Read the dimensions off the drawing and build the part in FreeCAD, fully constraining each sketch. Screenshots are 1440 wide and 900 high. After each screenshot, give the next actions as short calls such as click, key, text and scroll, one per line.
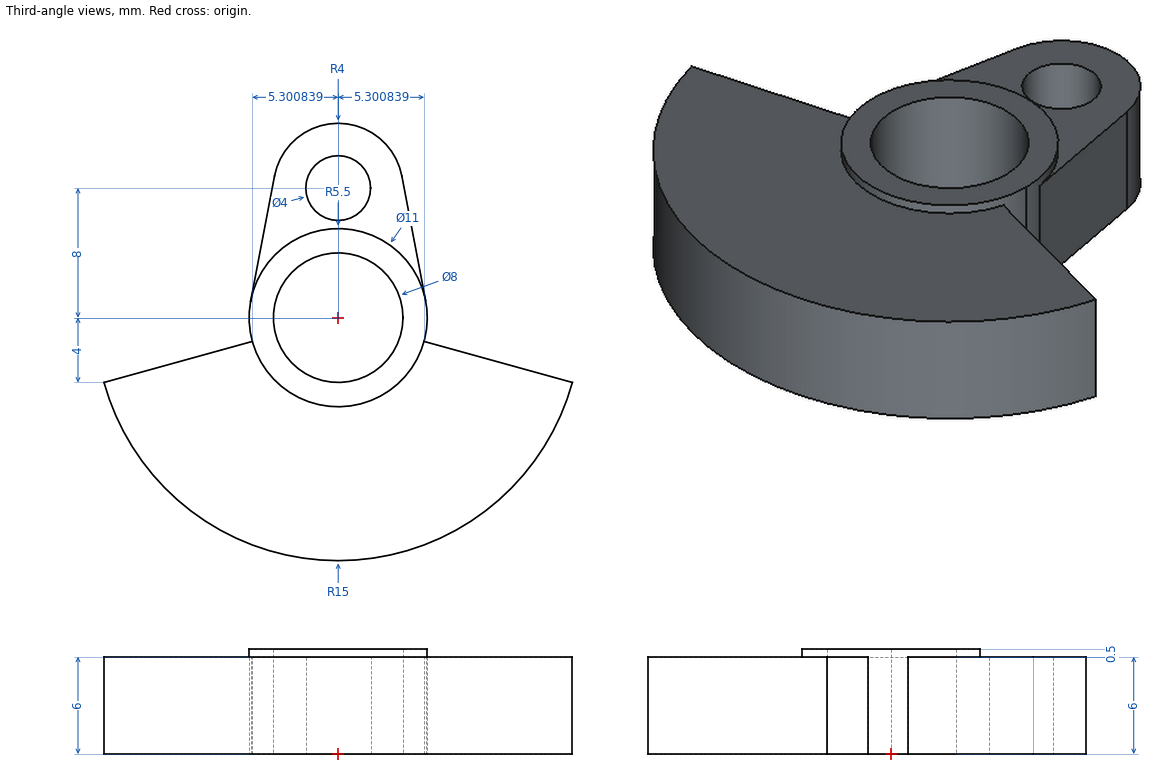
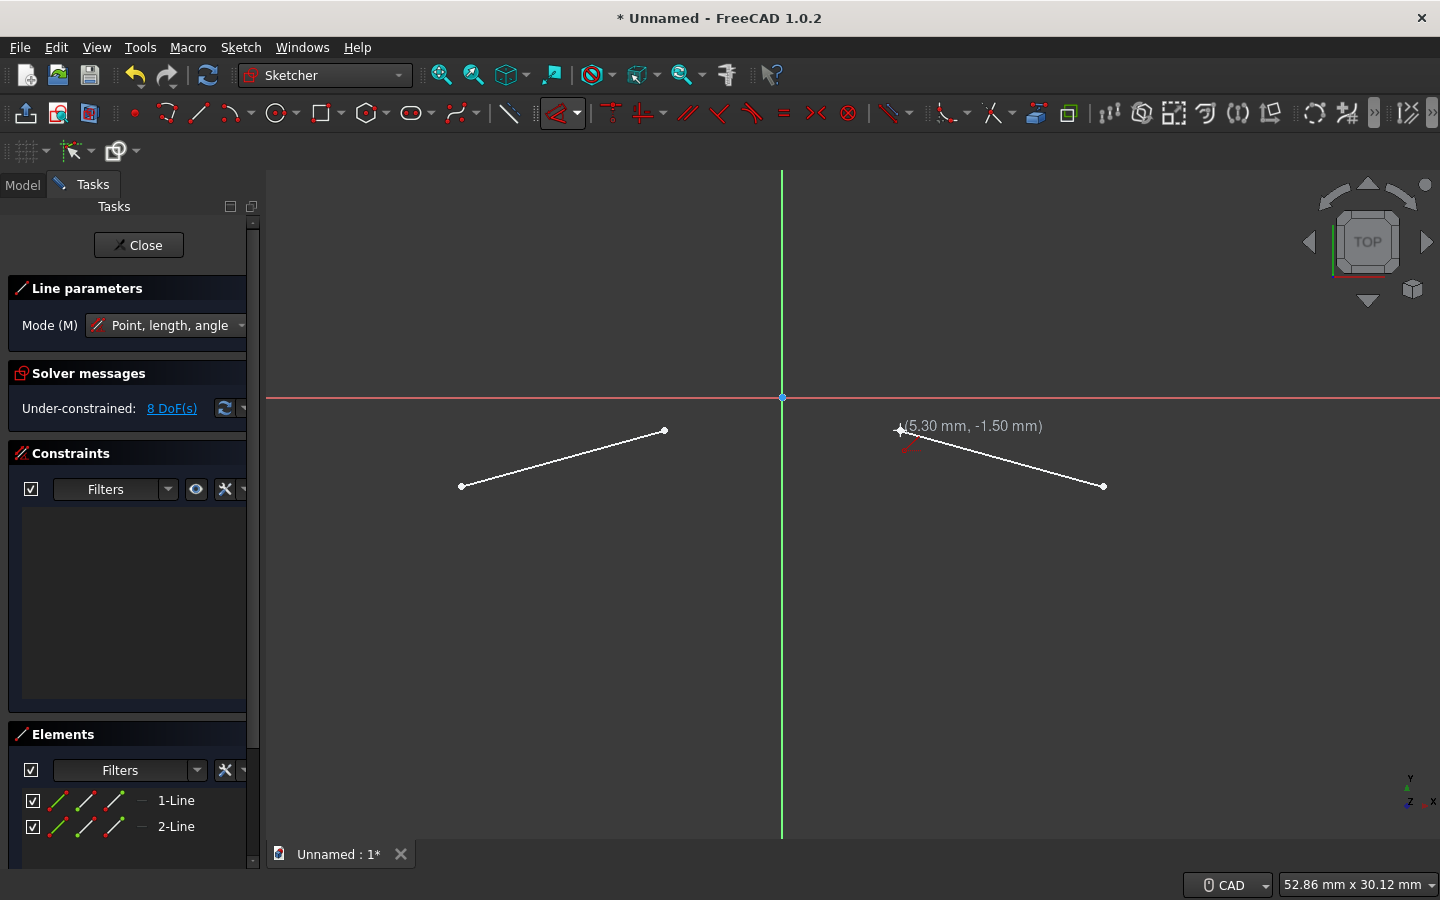
key(g)
key(3)
key(a)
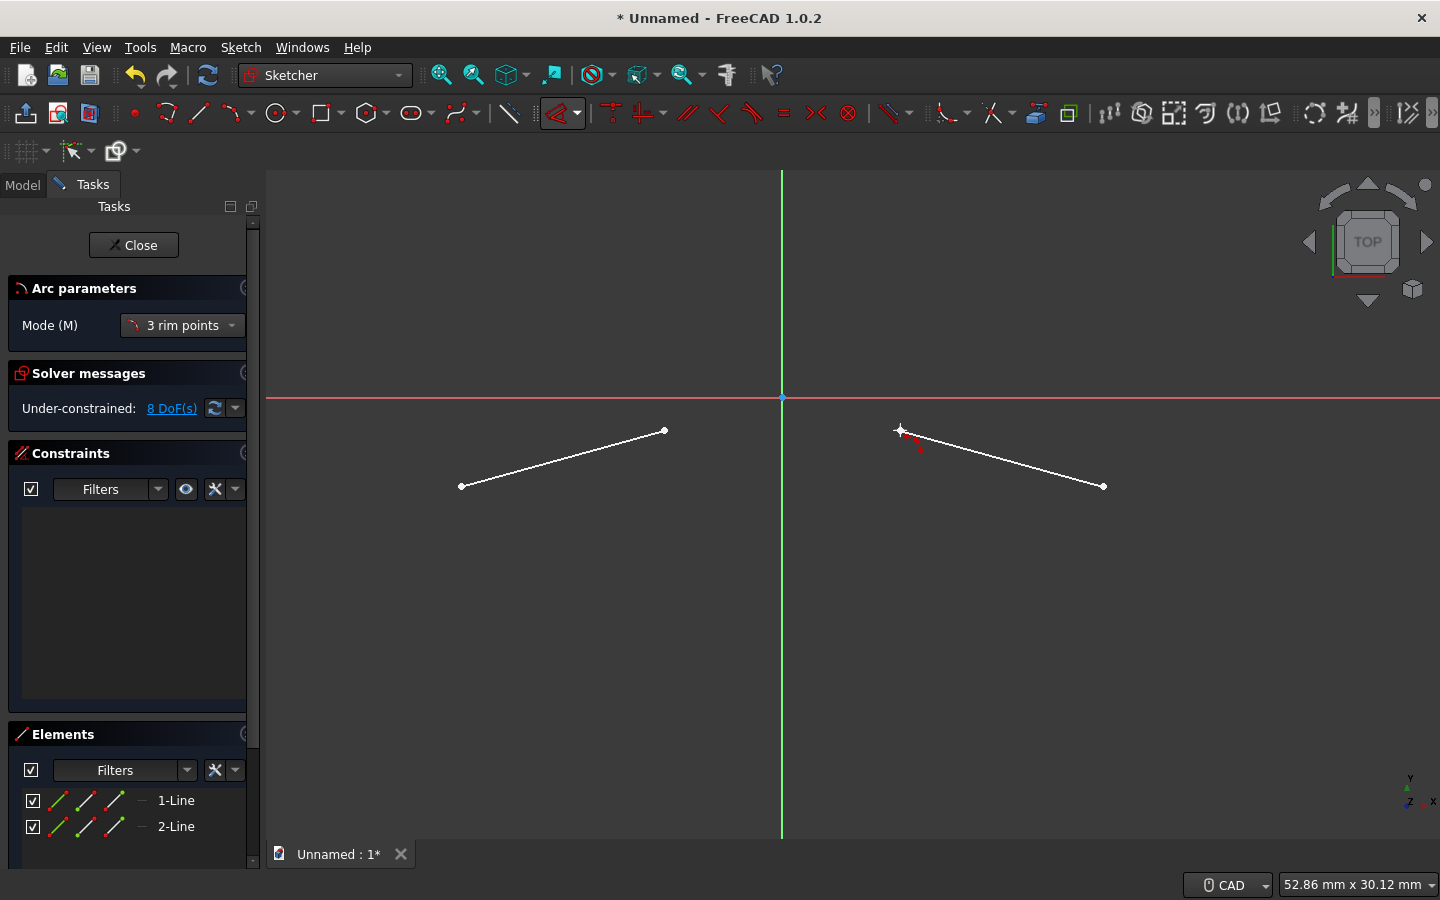
click(461, 487)
click(1103, 487)
click(696, 720)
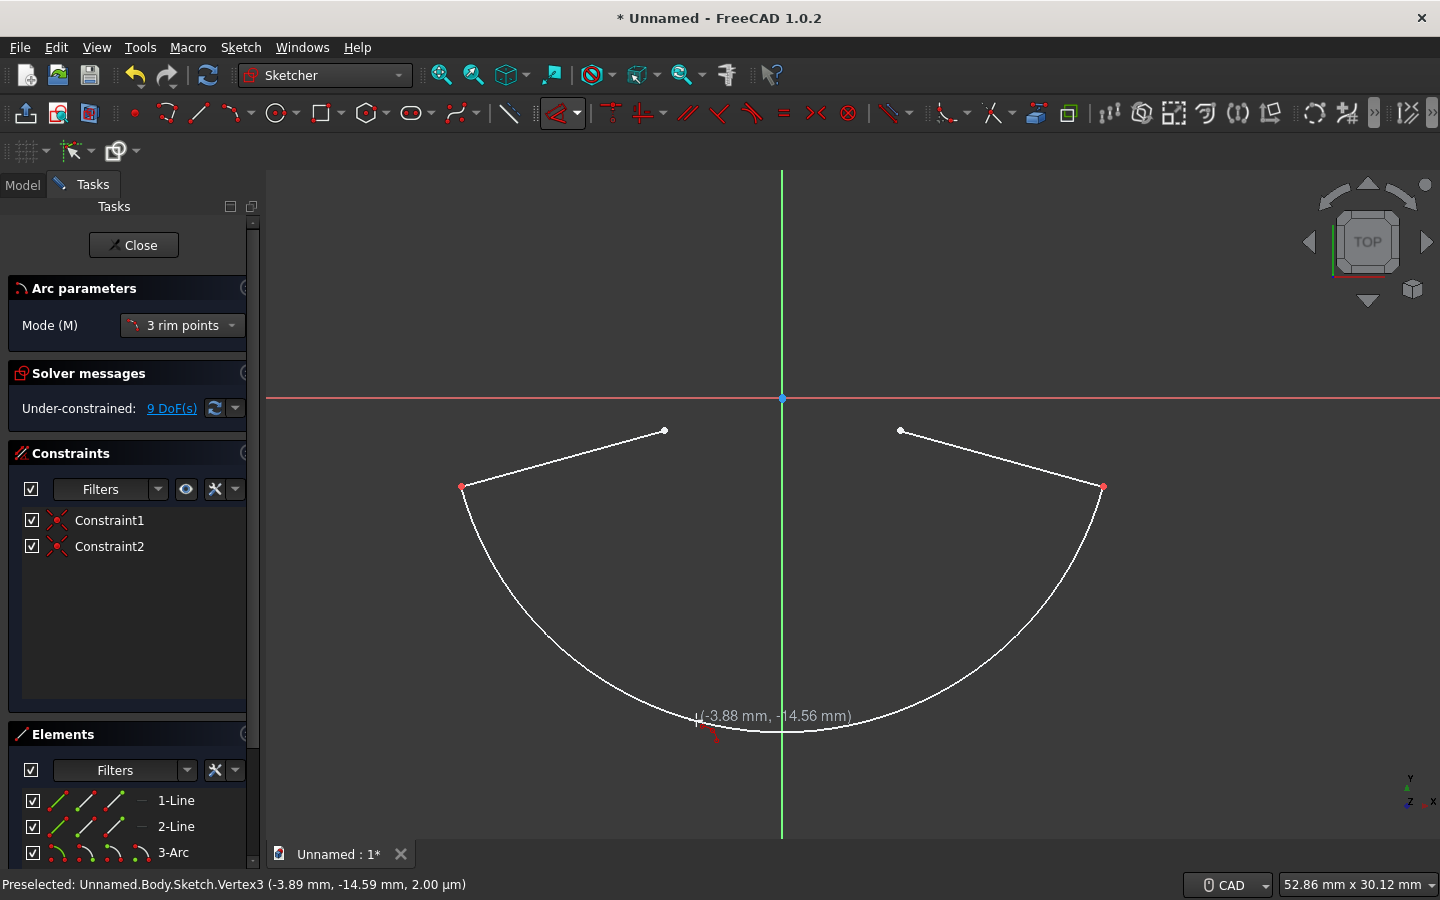
click(900, 431)
click(664, 431)
click(826, 284)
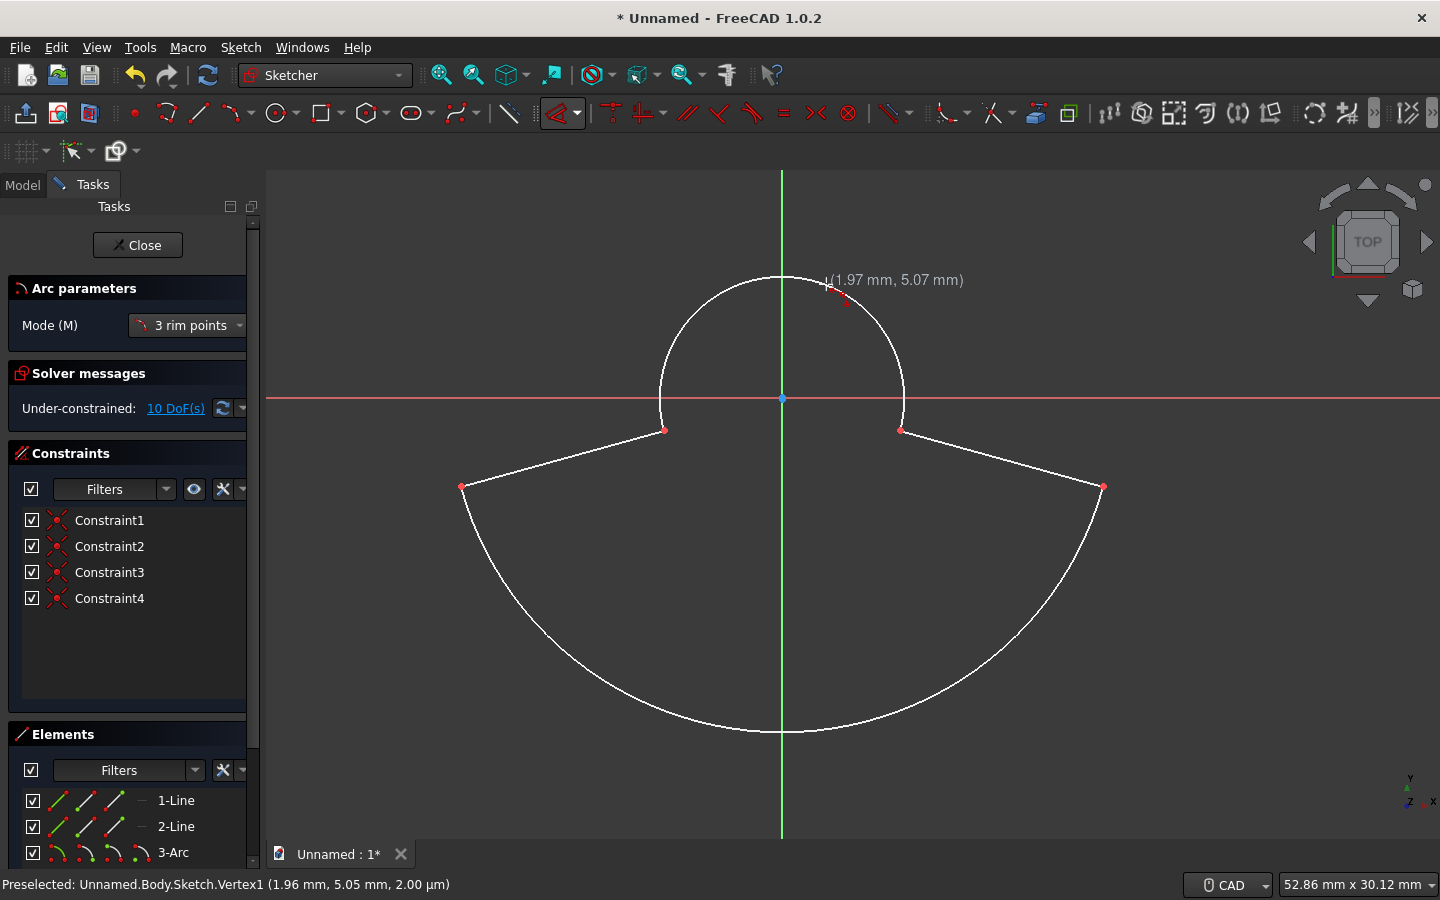
click(276, 114)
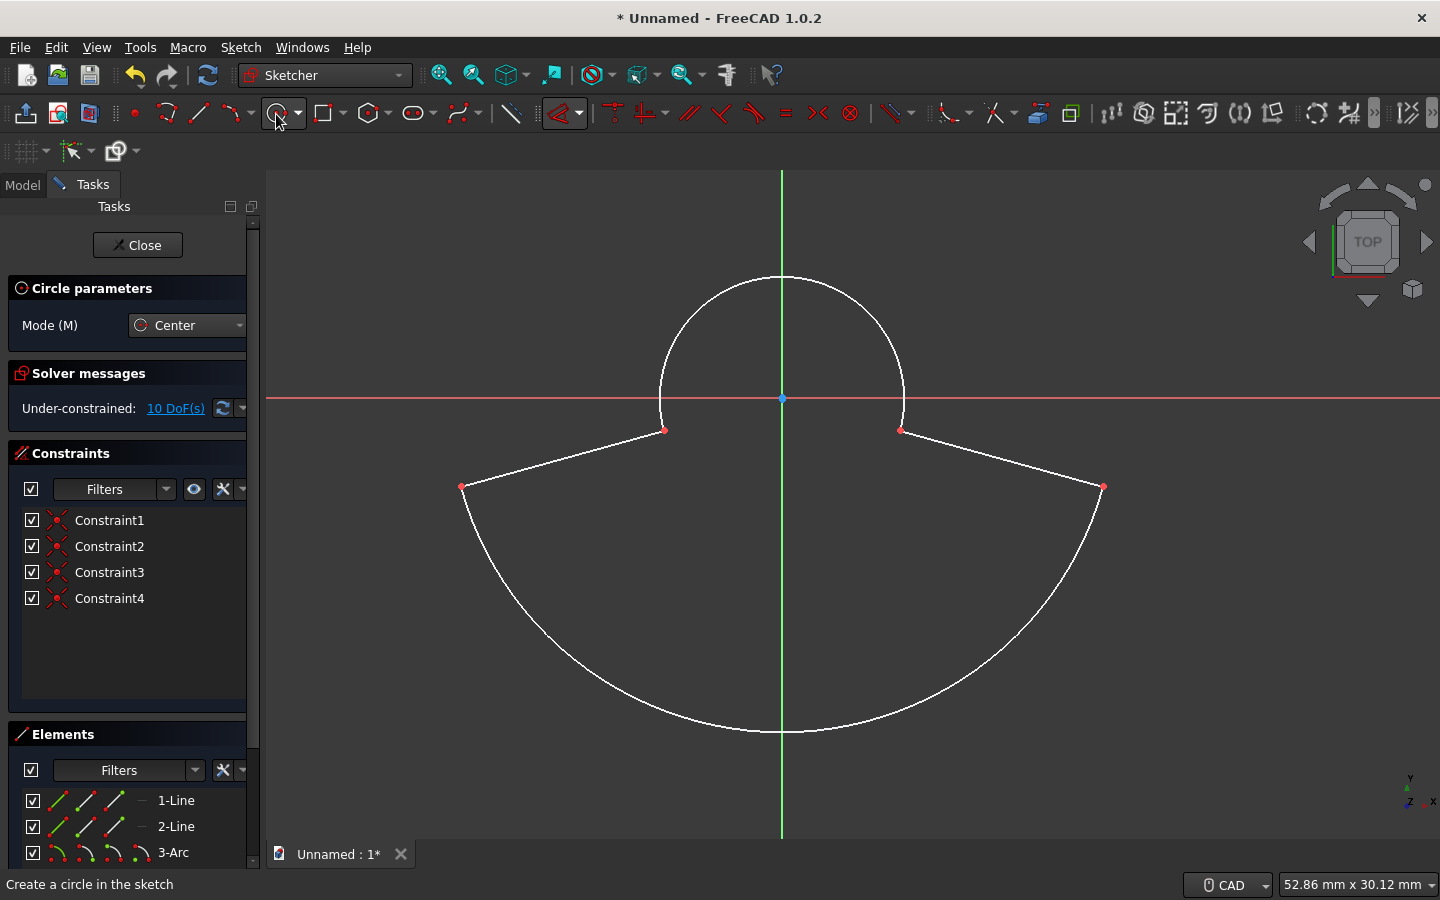
click(782, 398)
click(845, 335)
key(Escape)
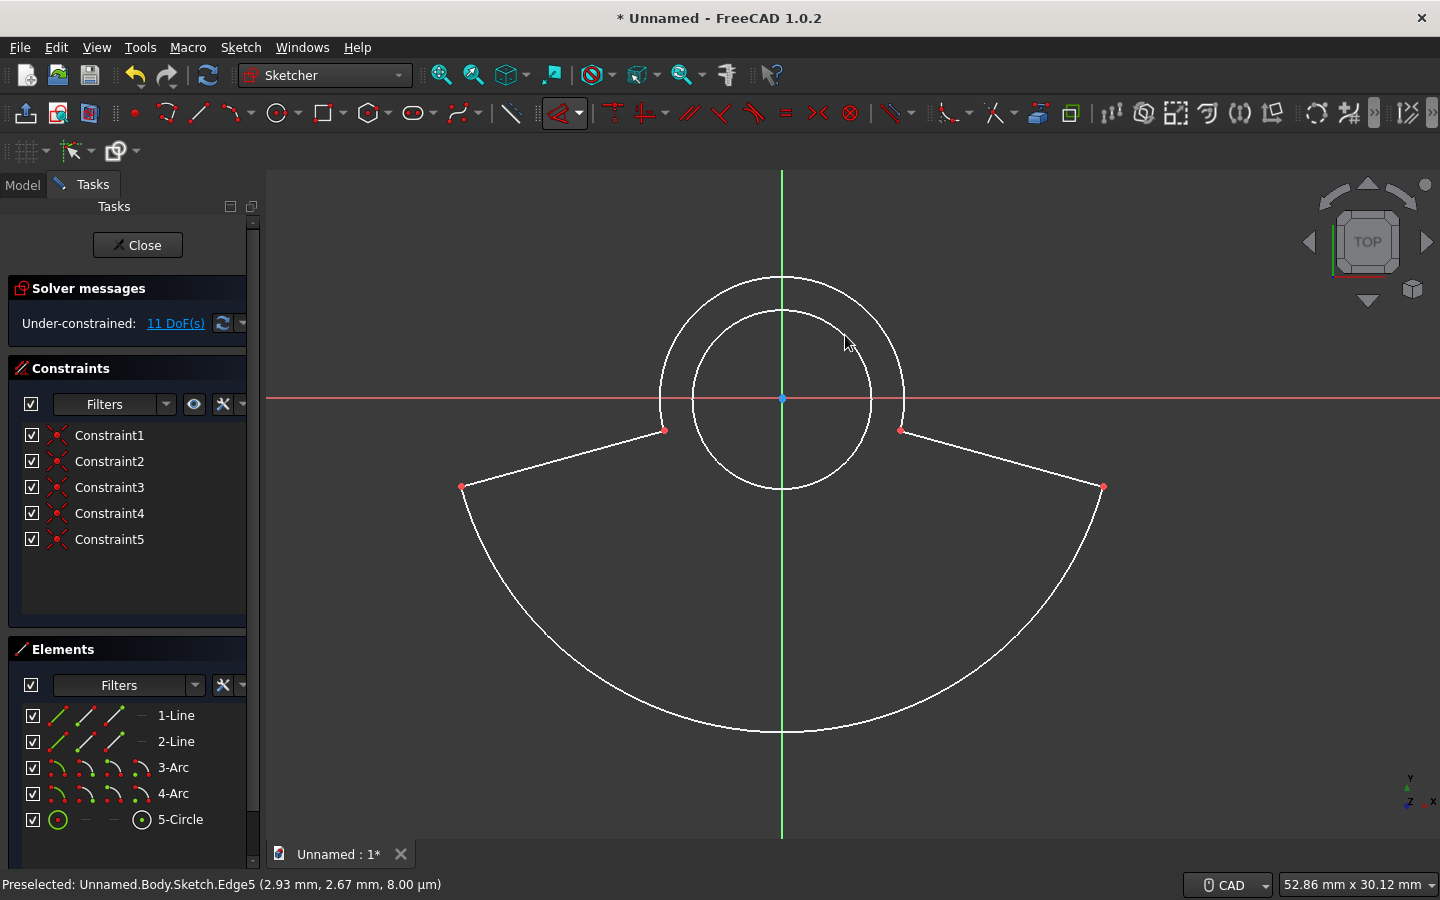
click(845, 336)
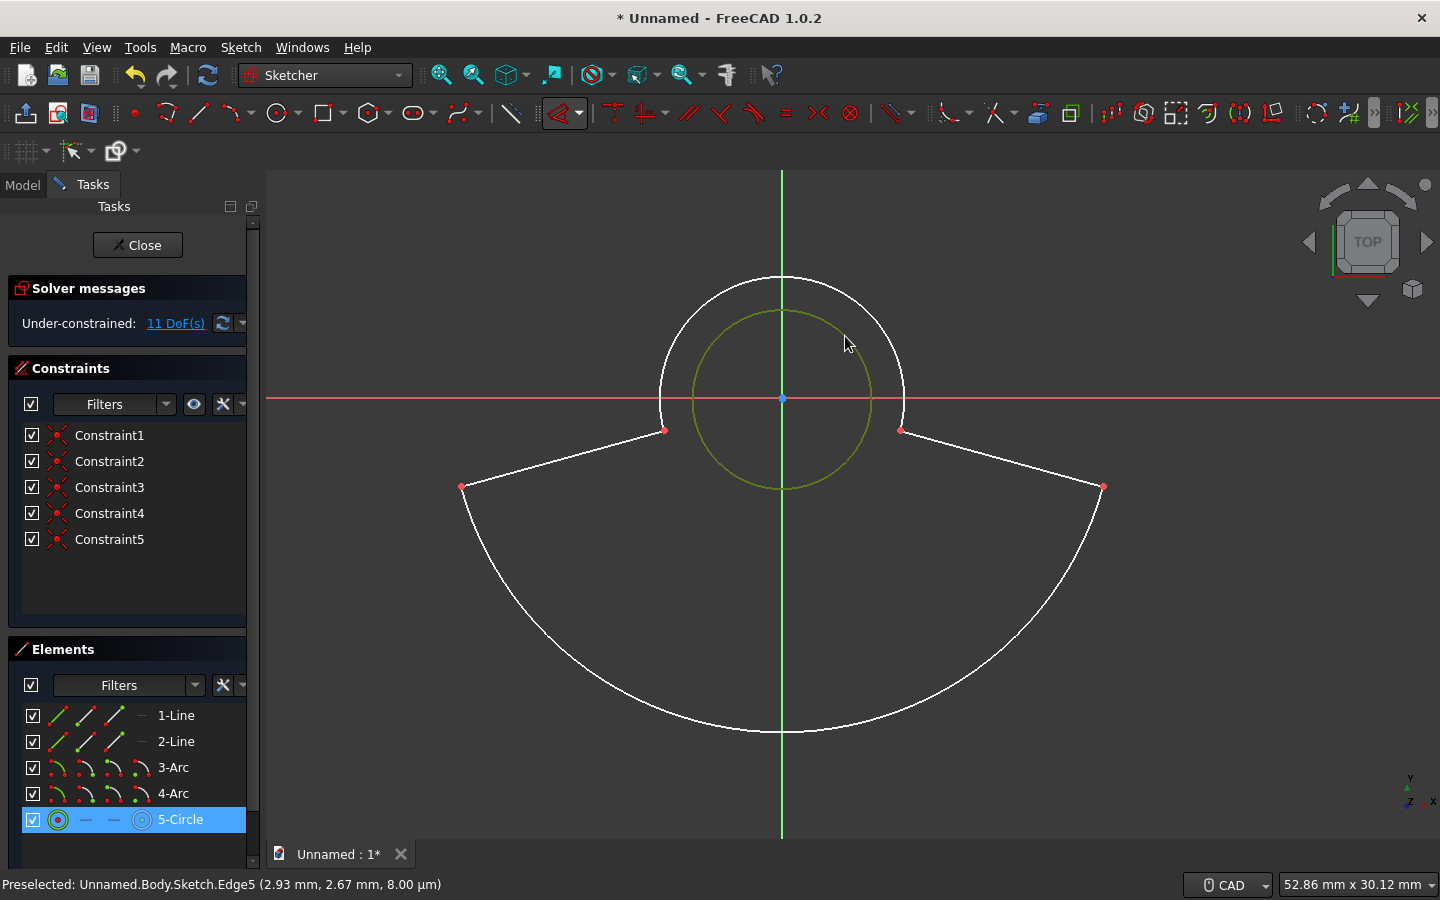
click(864, 308)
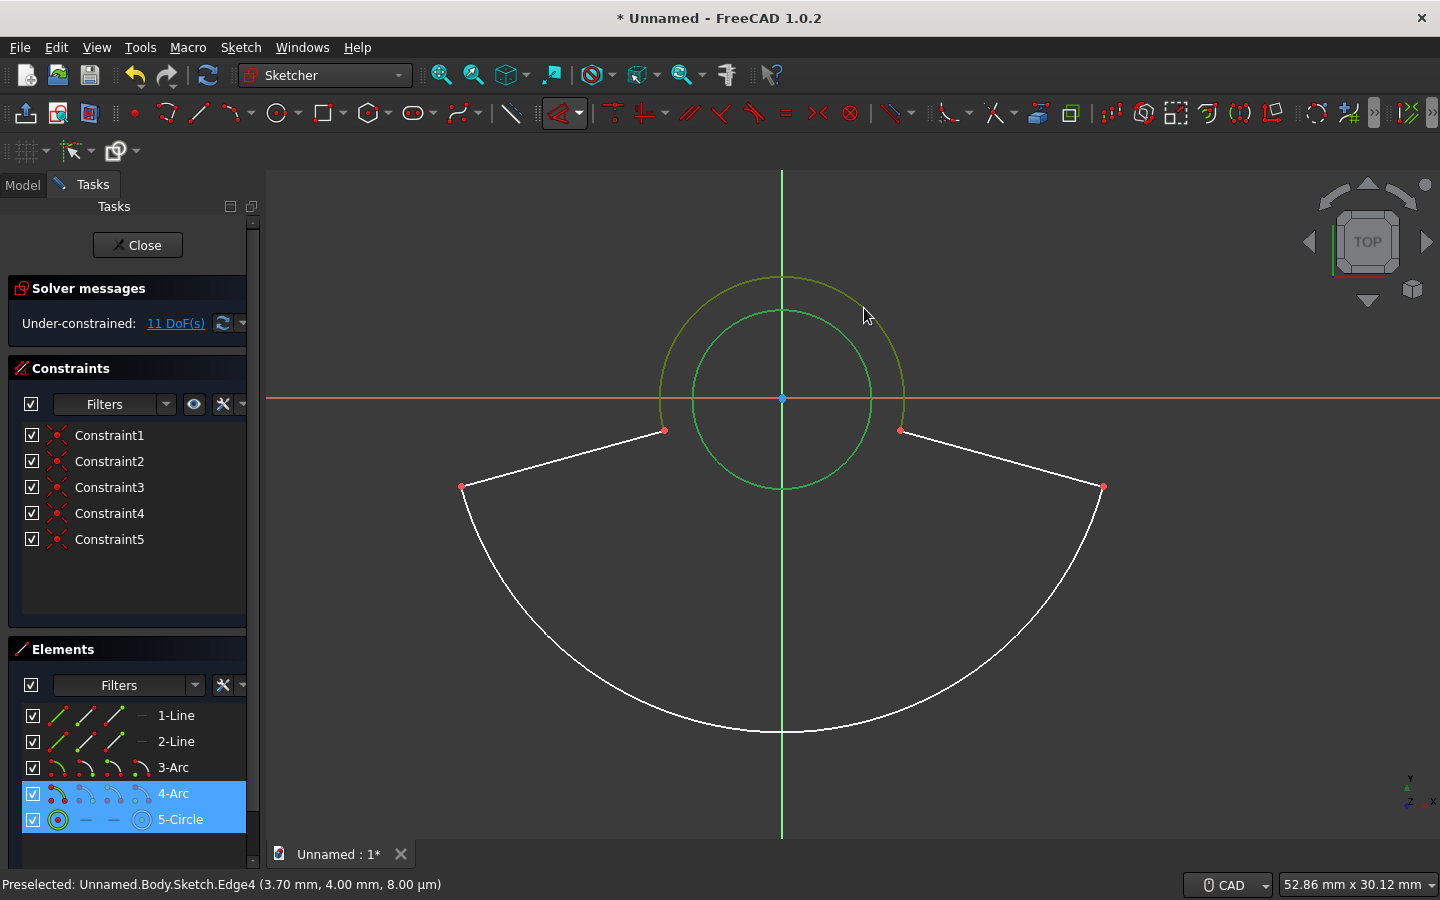
click(614, 114)